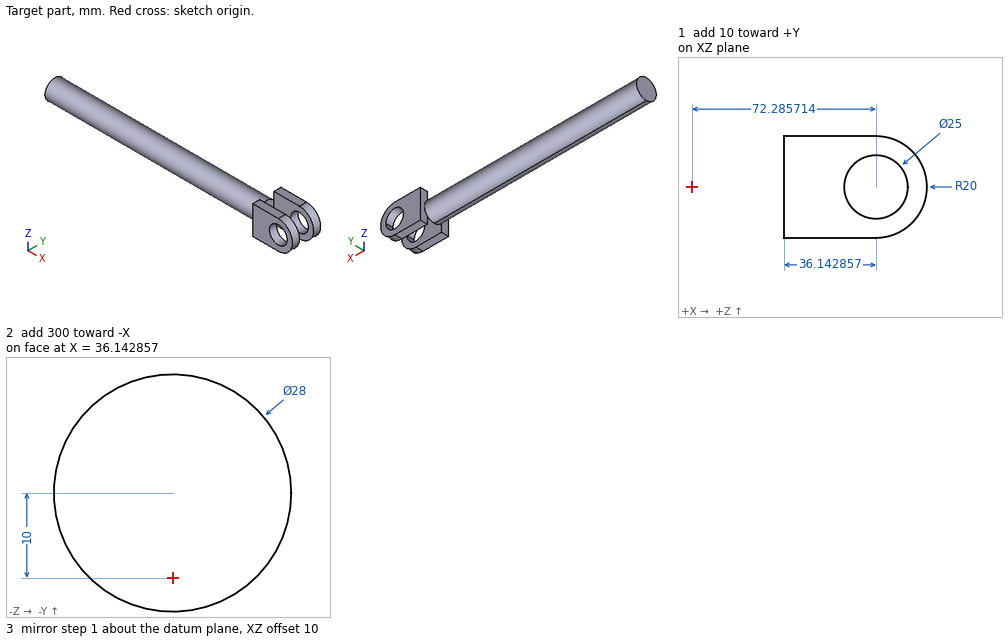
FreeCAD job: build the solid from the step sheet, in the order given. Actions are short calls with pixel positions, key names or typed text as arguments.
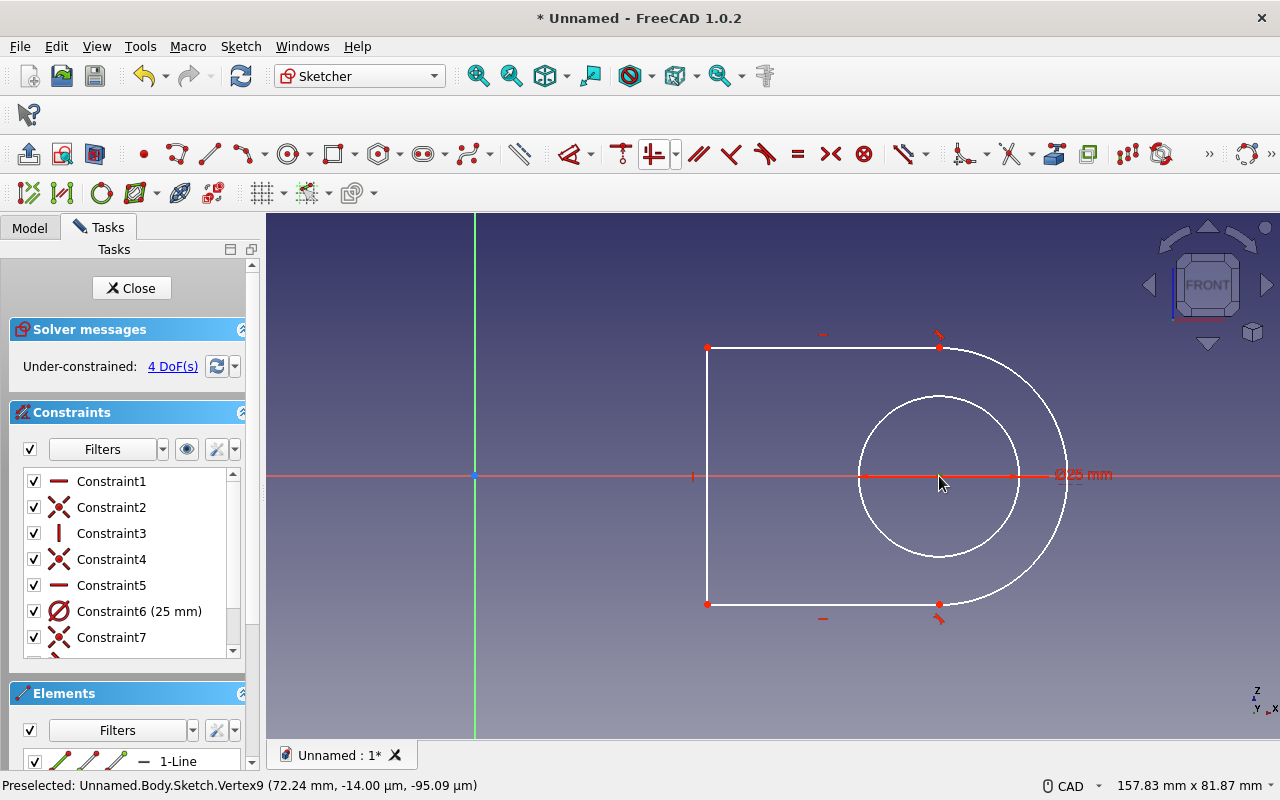
click(353, 476)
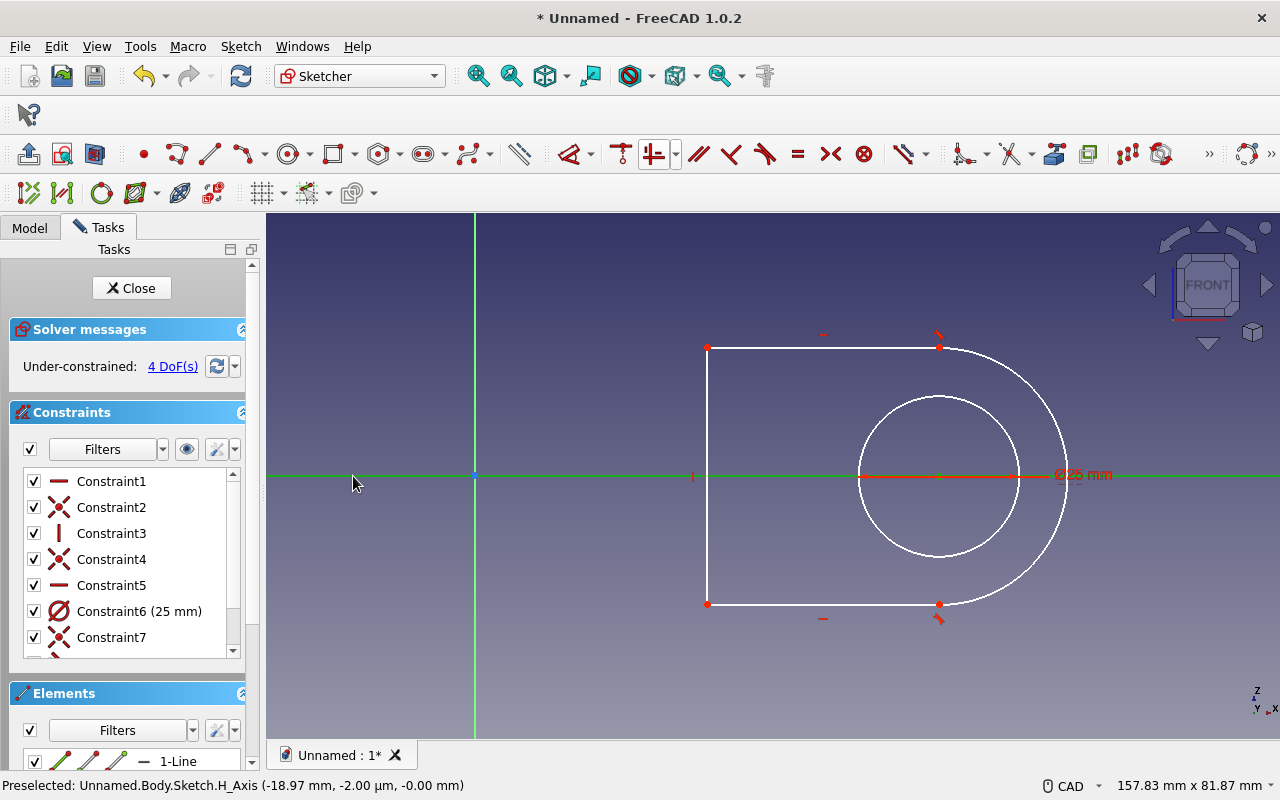
key(c)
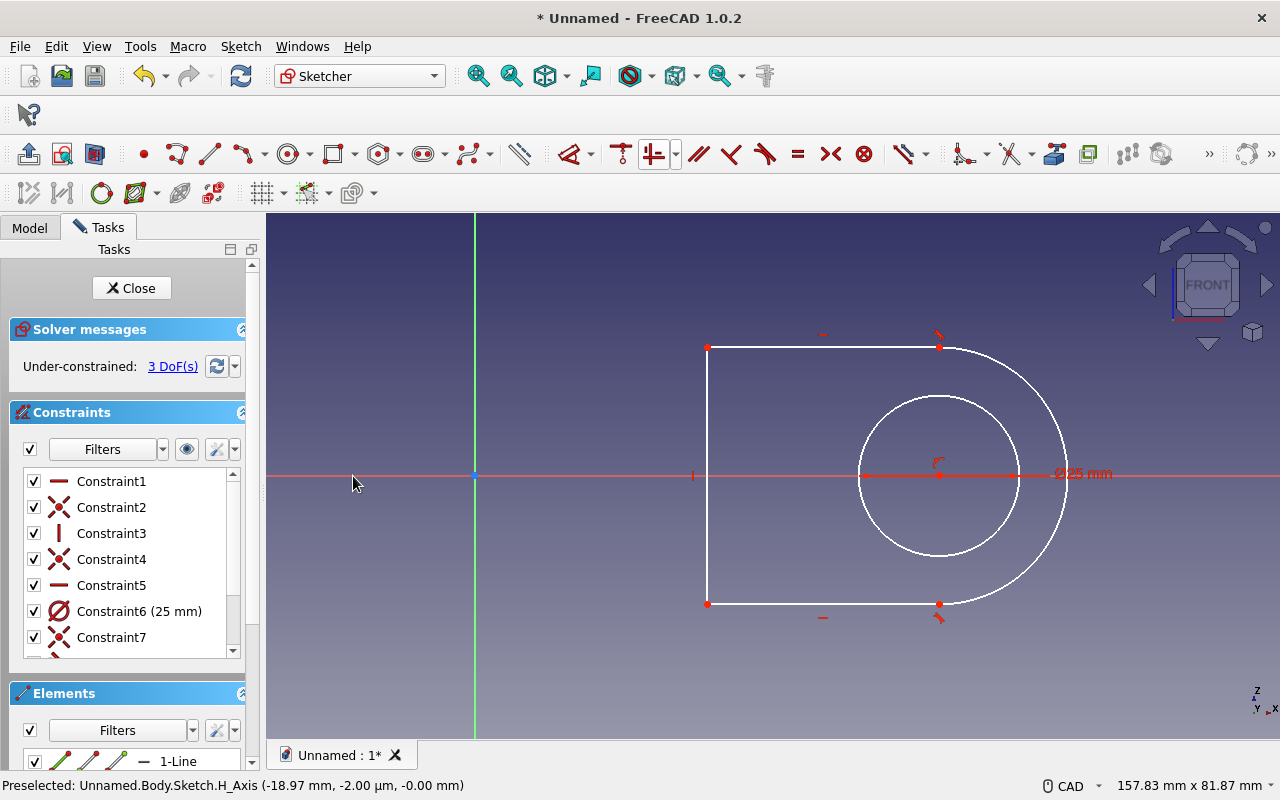
click(568, 154)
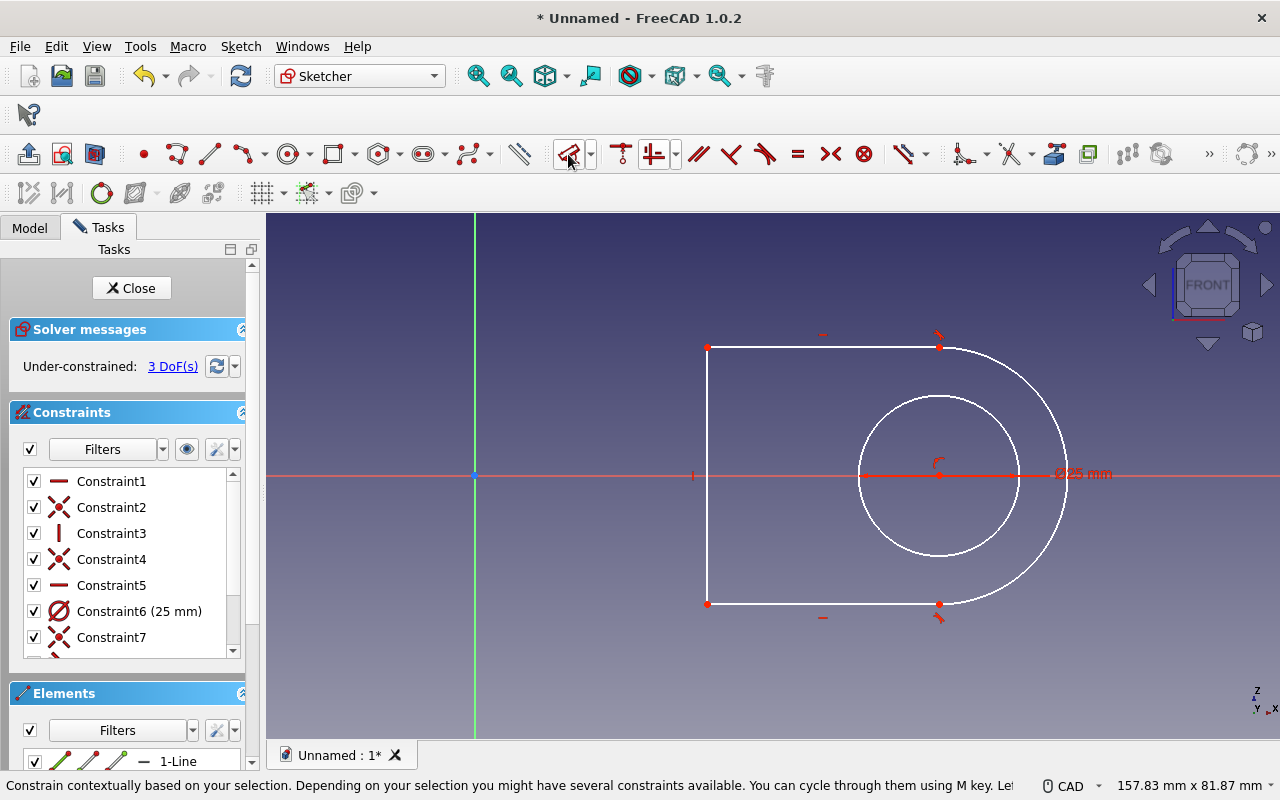
click(1043, 551)
click(1069, 570)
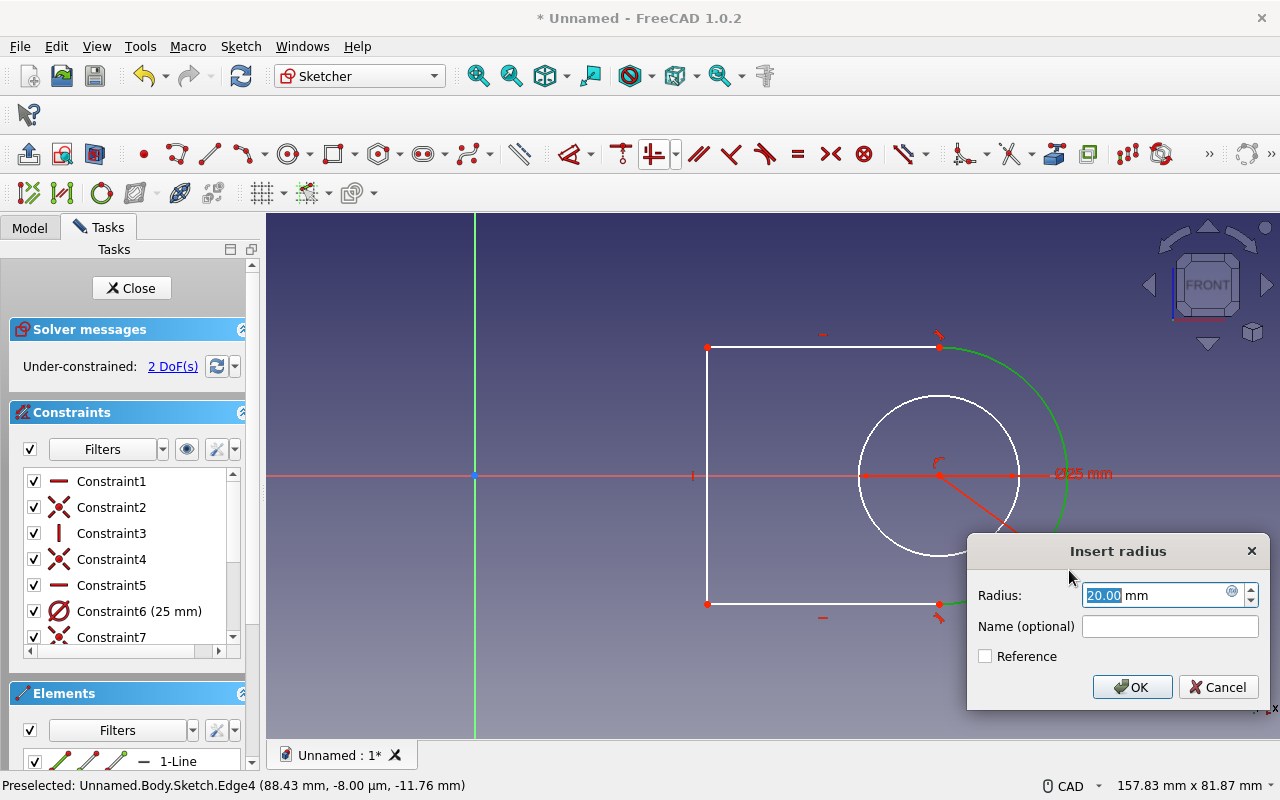
text(20)
key(Return)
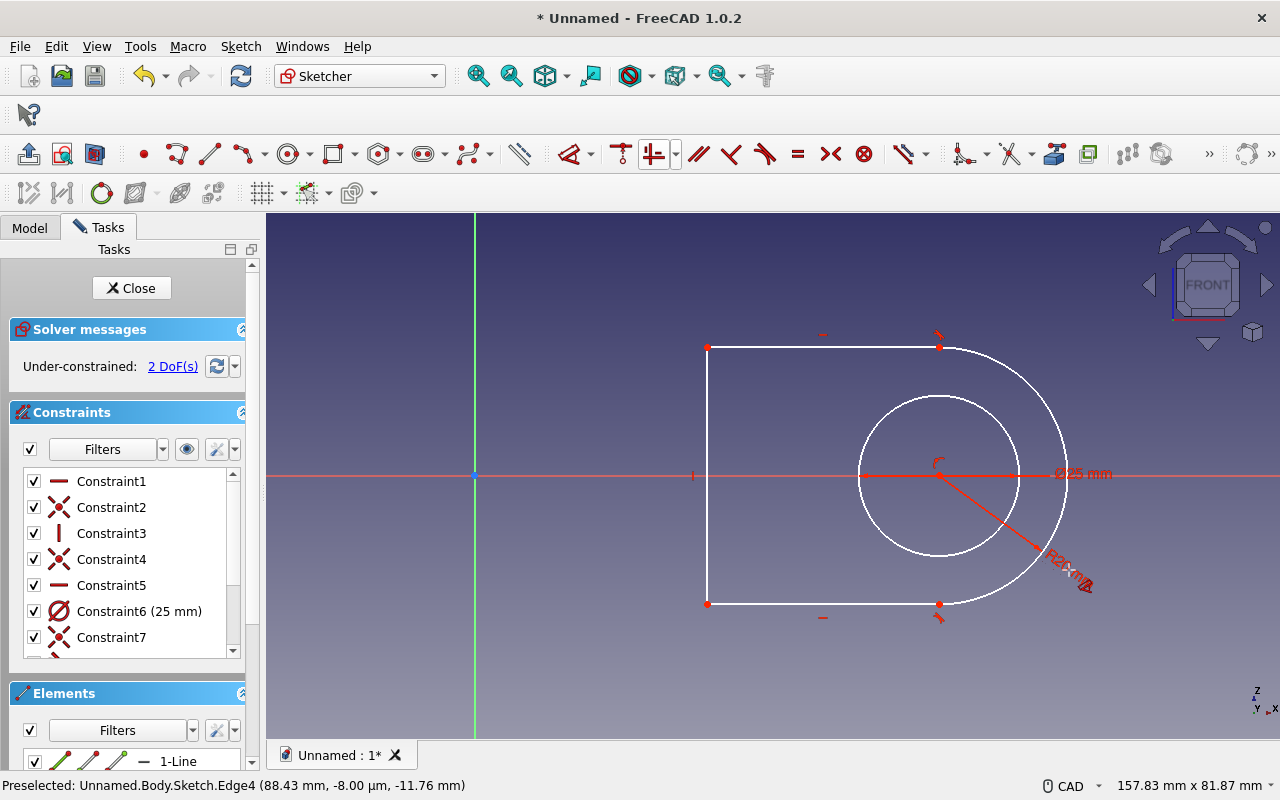
click(869, 604)
click(823, 638)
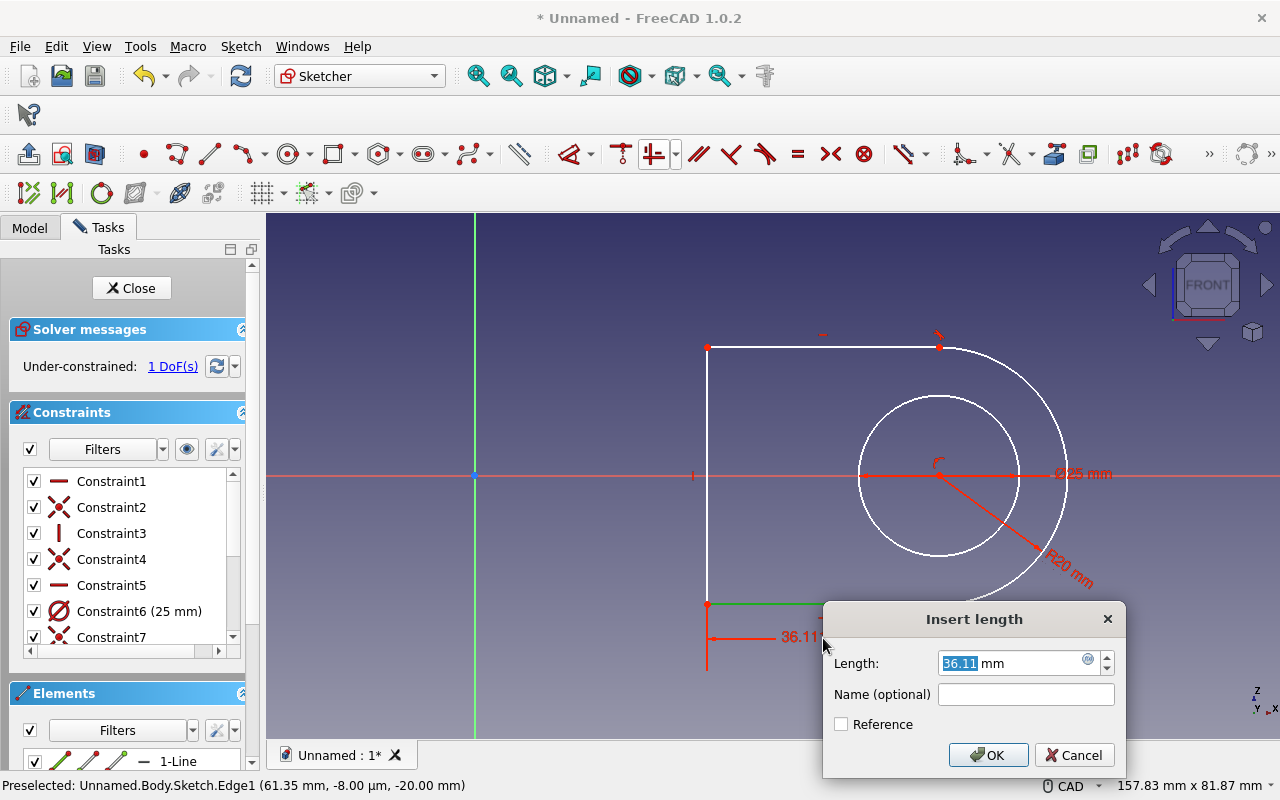
text(36.142857)
key(Return)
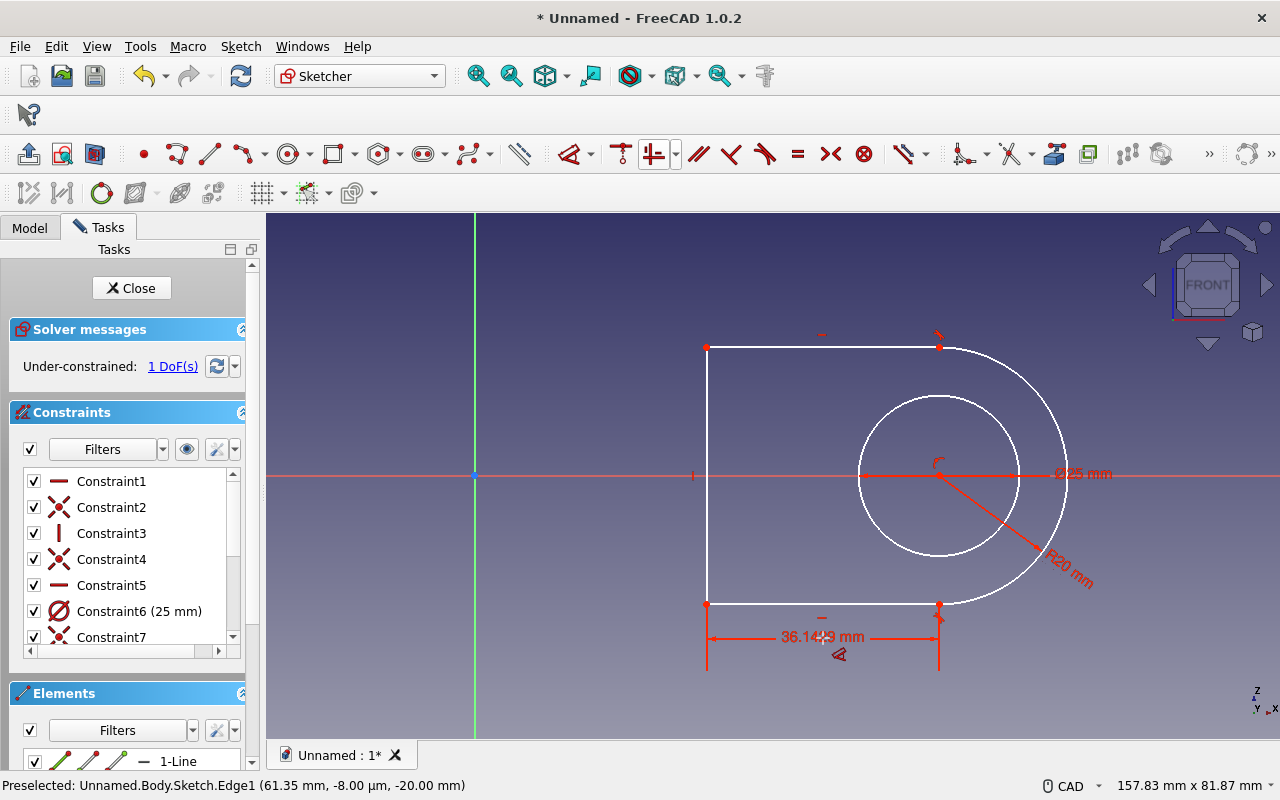
click(939, 476)
click(600, 510)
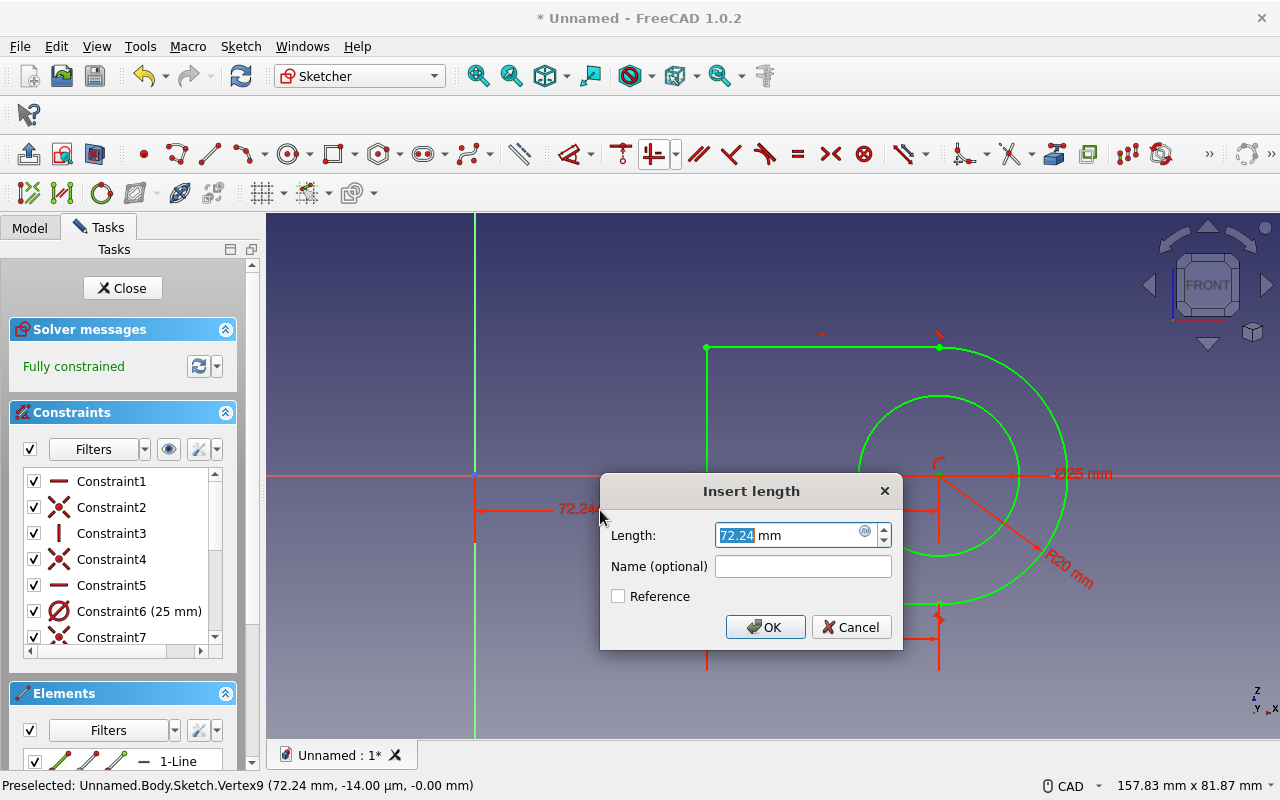
text(72.285714)
key(Return)
key(Escape)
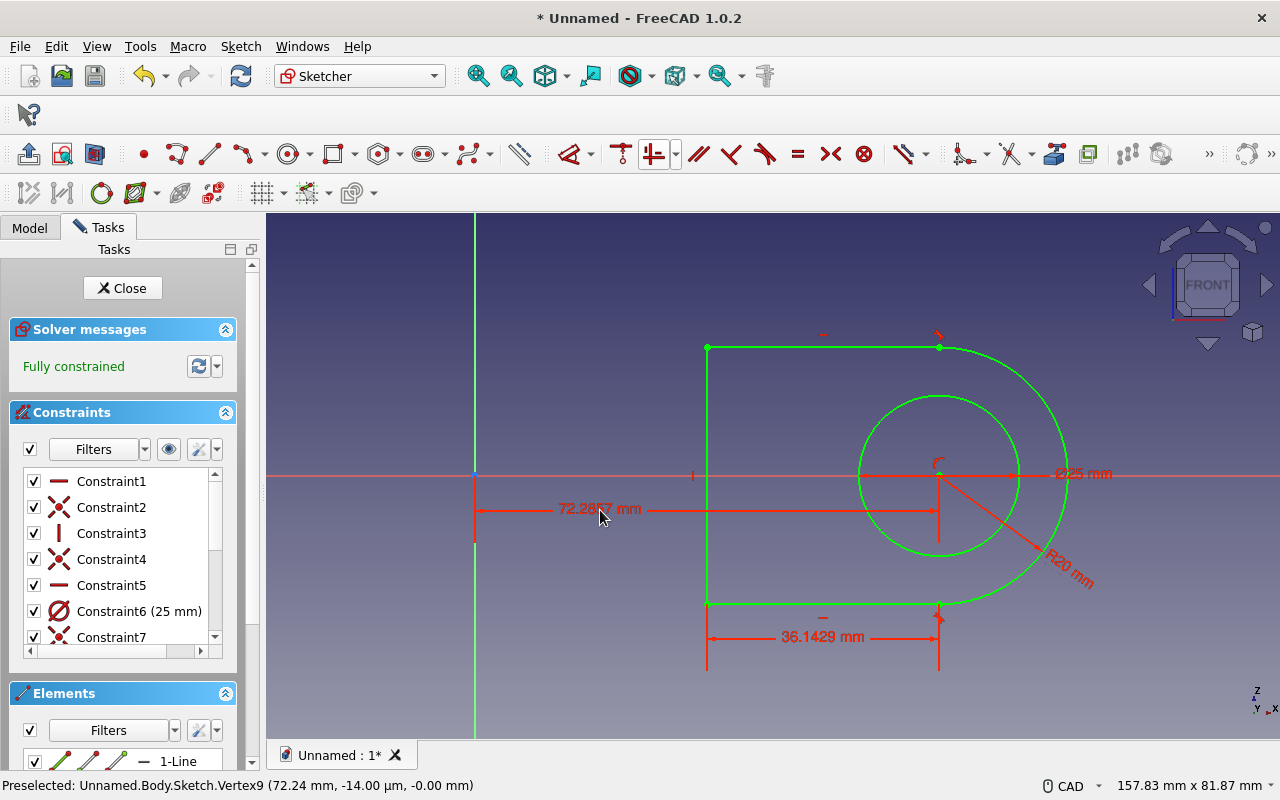
click(123, 288)